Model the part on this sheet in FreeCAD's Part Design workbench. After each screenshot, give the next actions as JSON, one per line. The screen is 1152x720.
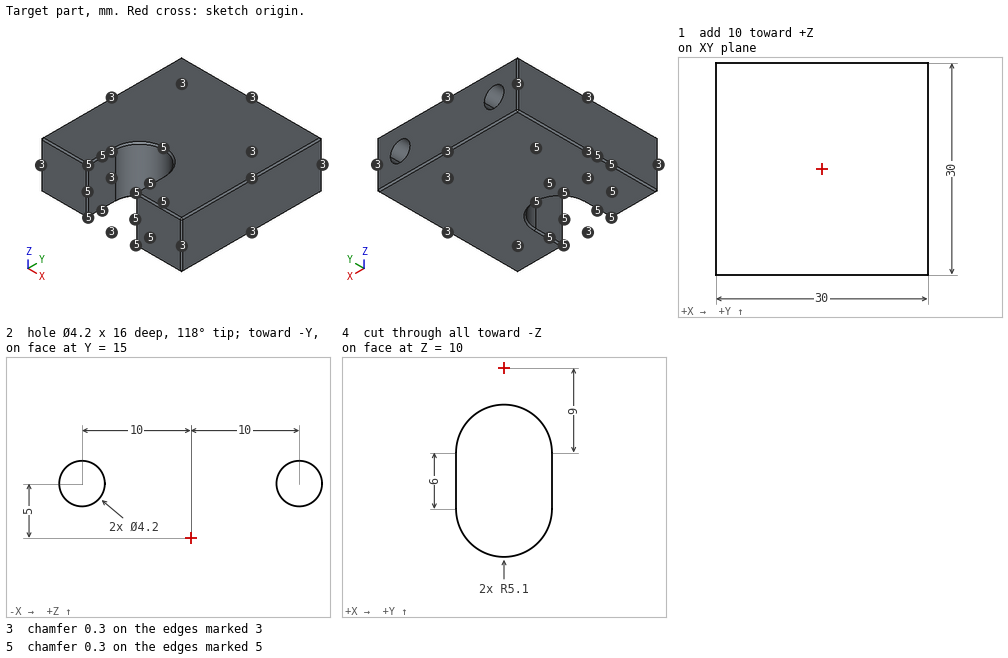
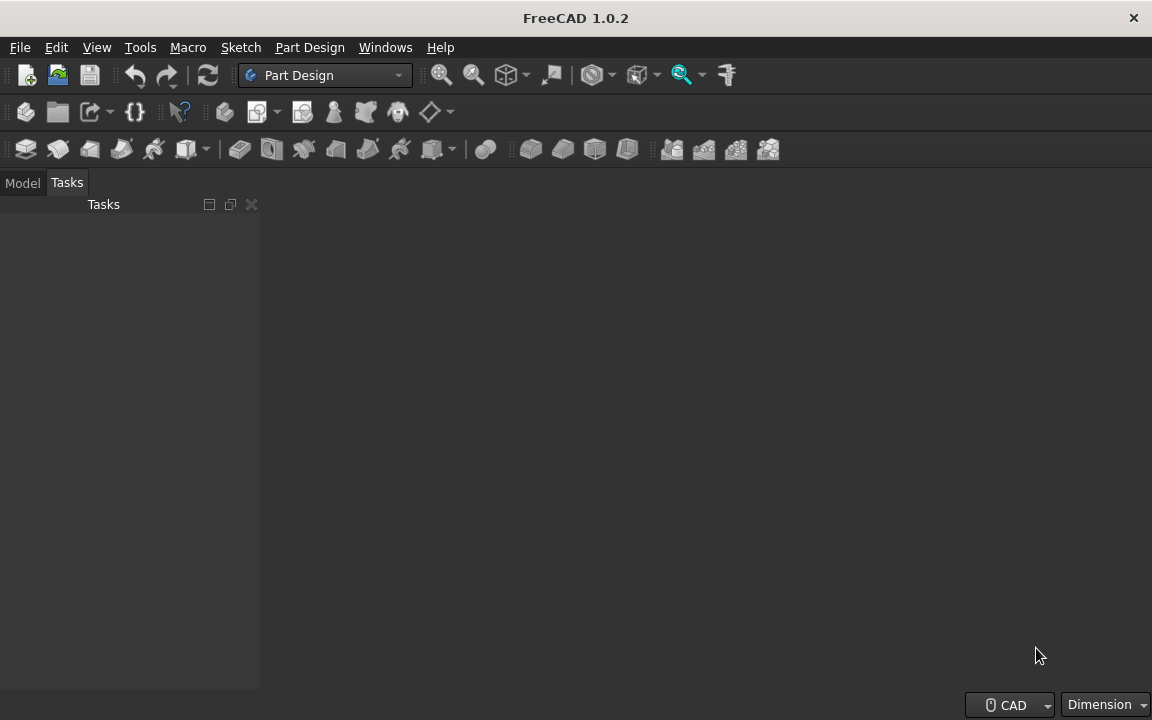
{"action": "left_click", "coordinate": [26, 76]}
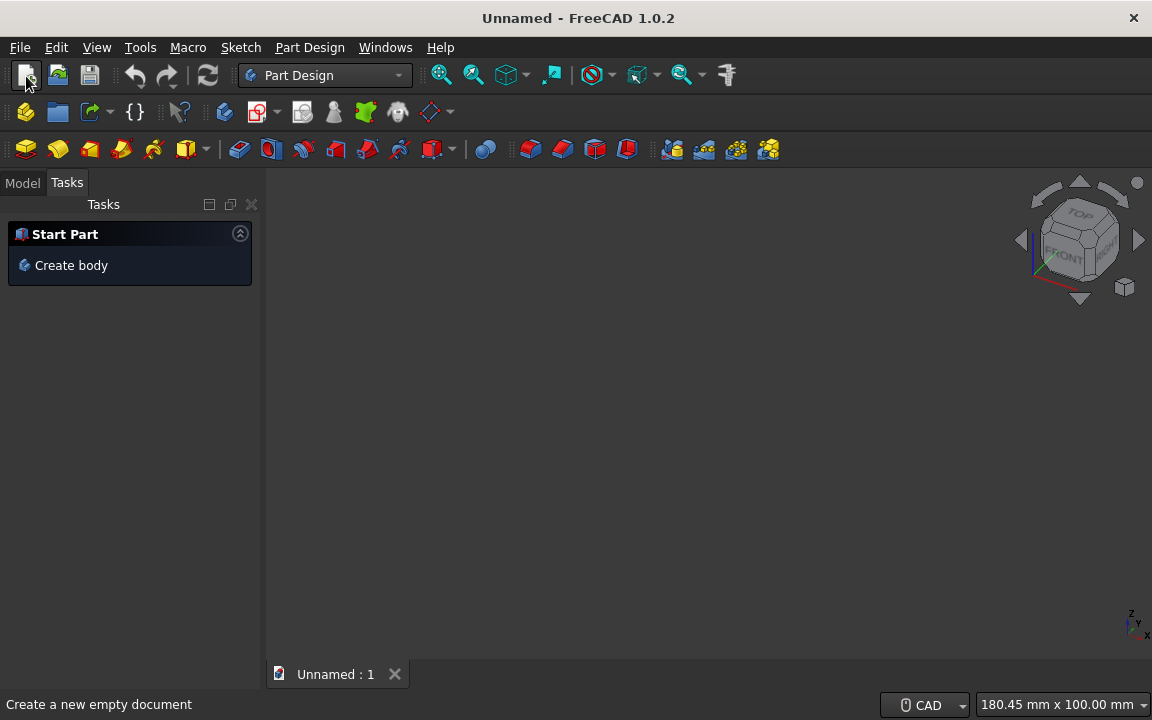
{"action": "left_click", "coordinate": [258, 112]}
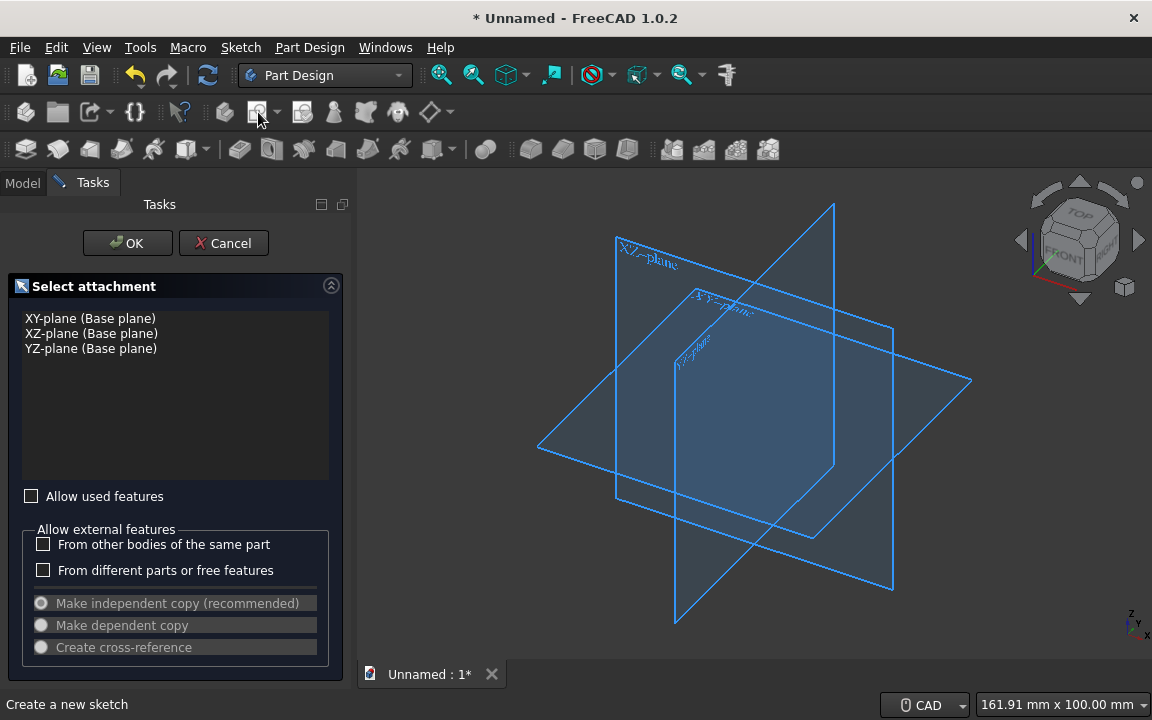
{"action": "left_click", "coordinate": [82, 318]}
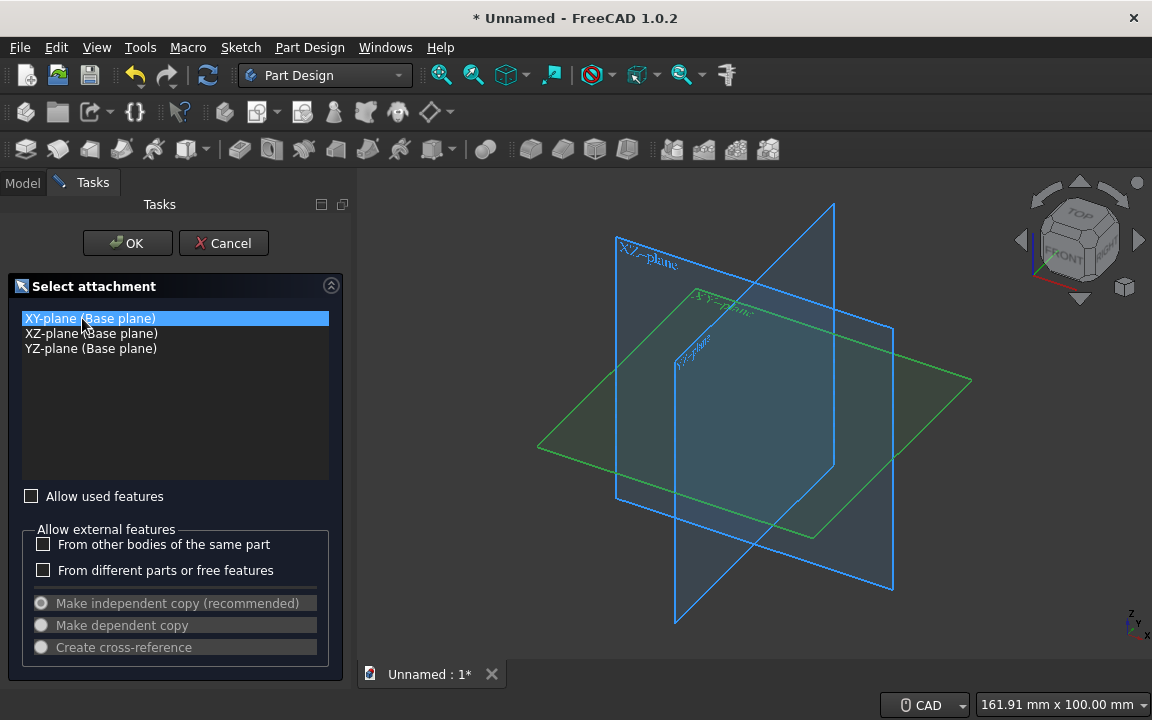
{"action": "left_click", "coordinate": [128, 243]}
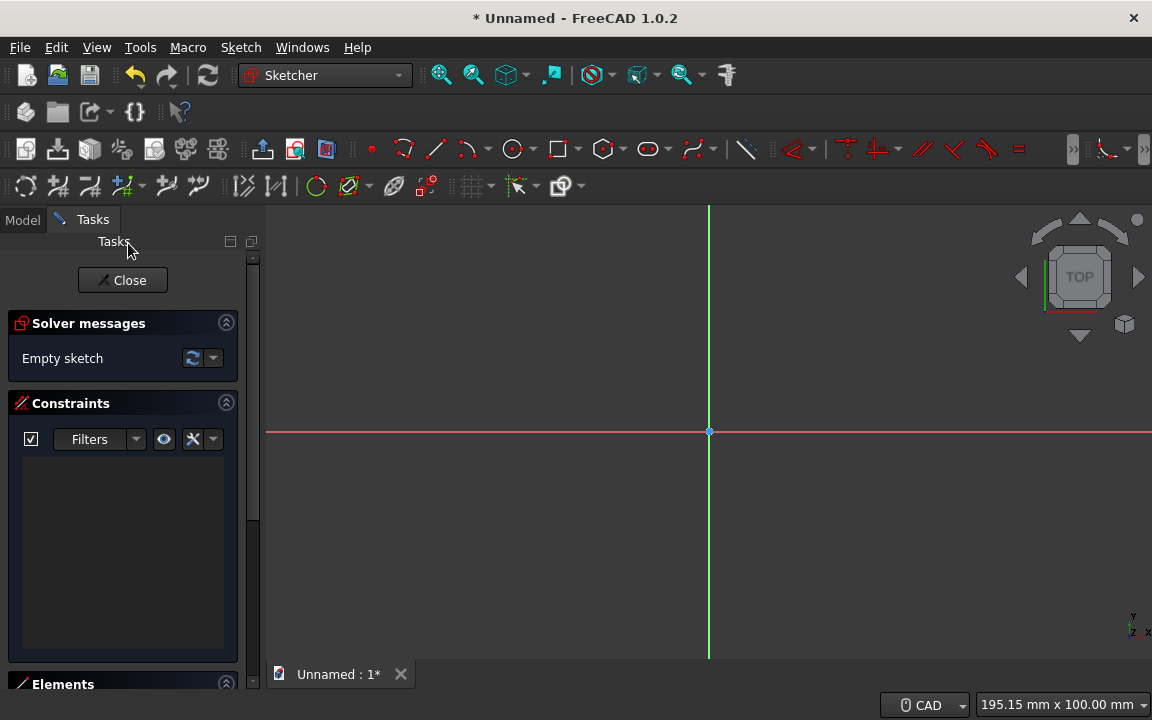
{"action": "scroll", "coordinate": [765, 432], "scroll_direction": "up", "scroll_amount": 4}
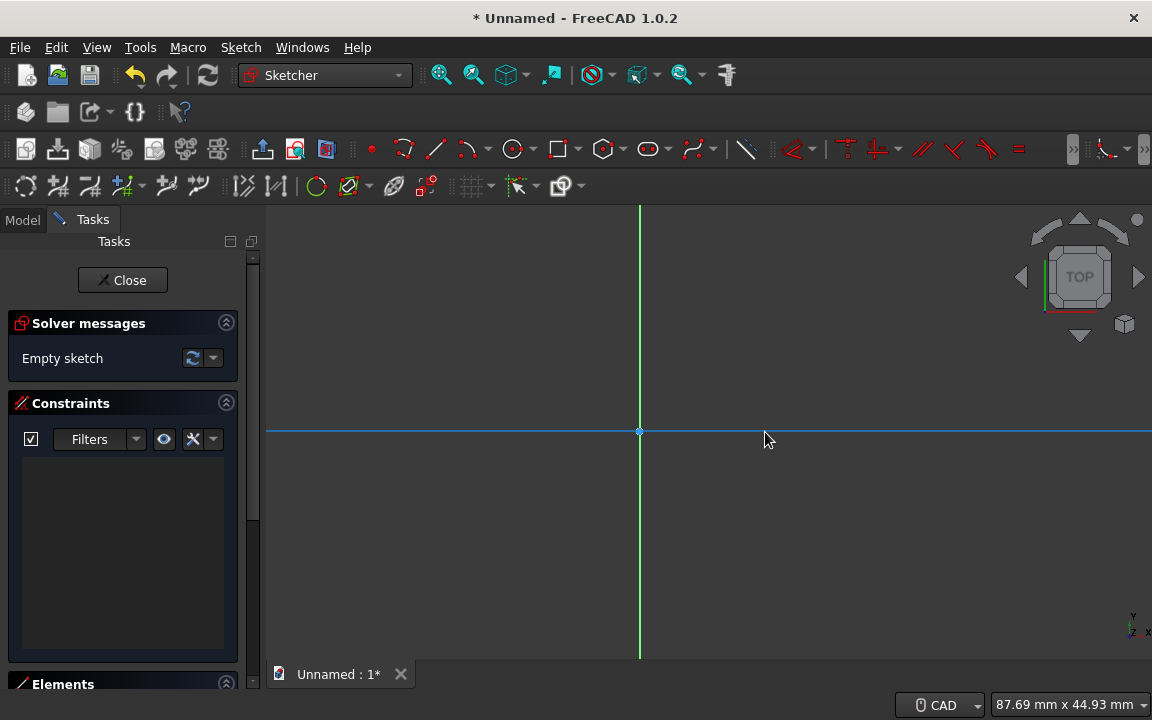
{"action": "left_click", "coordinate": [580, 150]}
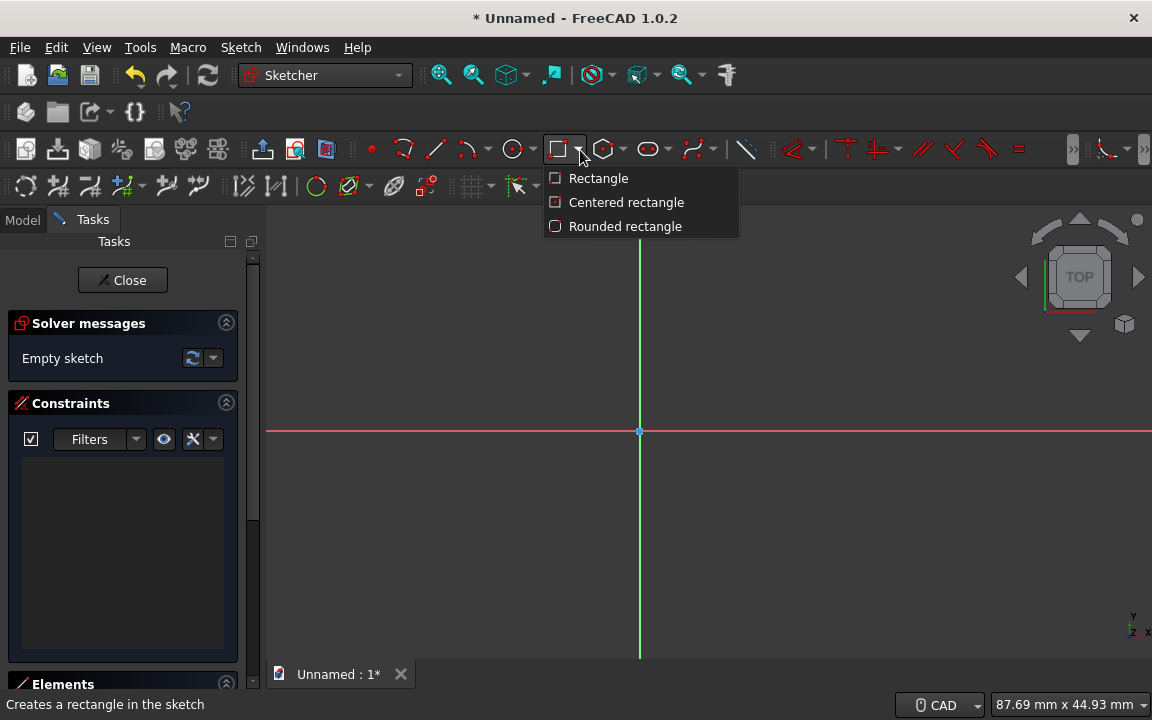
{"action": "left_click", "coordinate": [642, 202]}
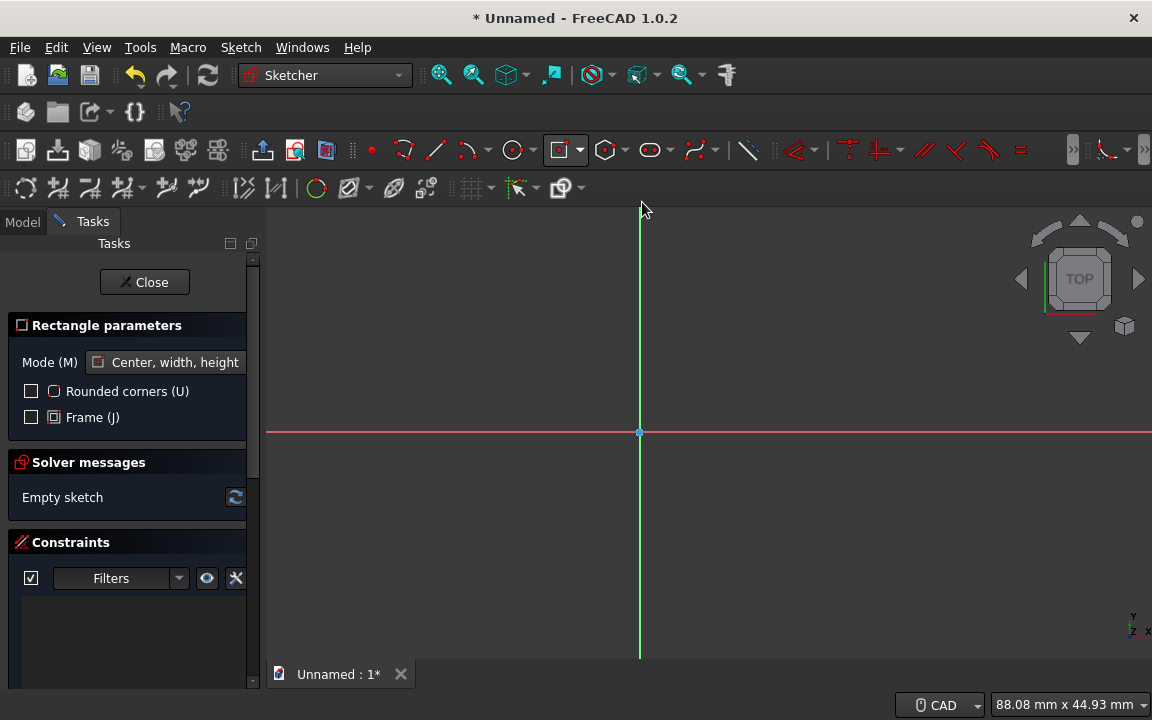
{"action": "left_click", "coordinate": [640, 432]}
{"action": "left_click", "coordinate": [791, 281]}
{"action": "key", "text": "Escape"}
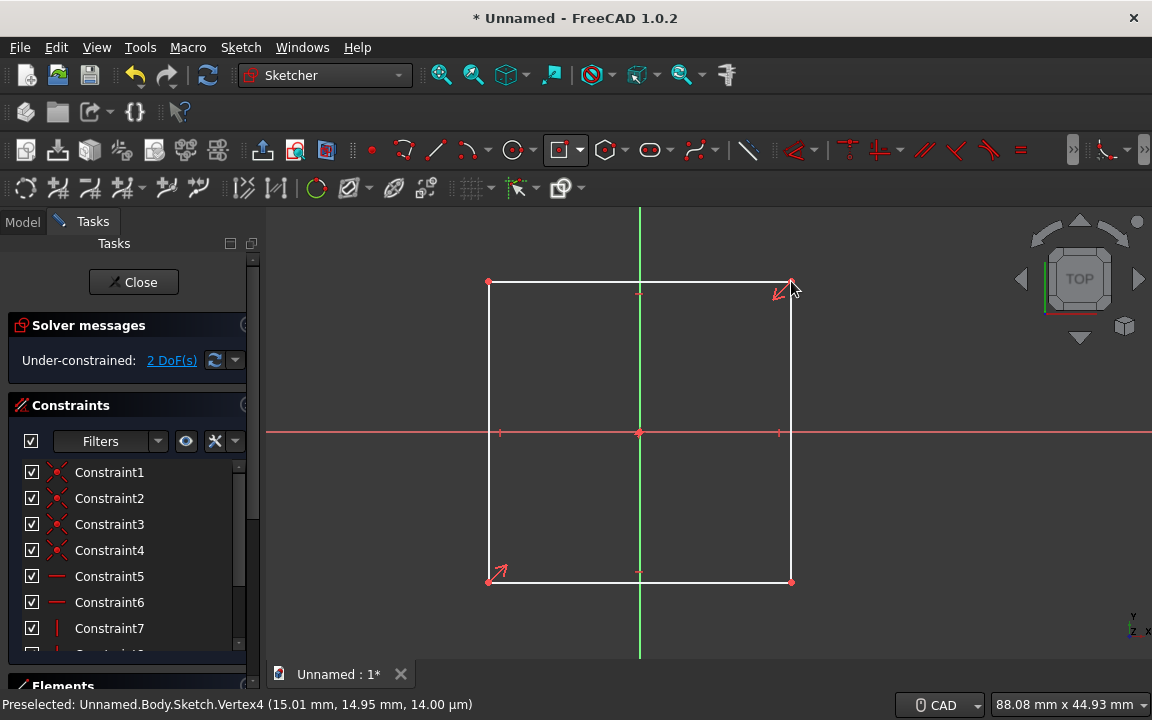
{"action": "left_click", "coordinate": [794, 150]}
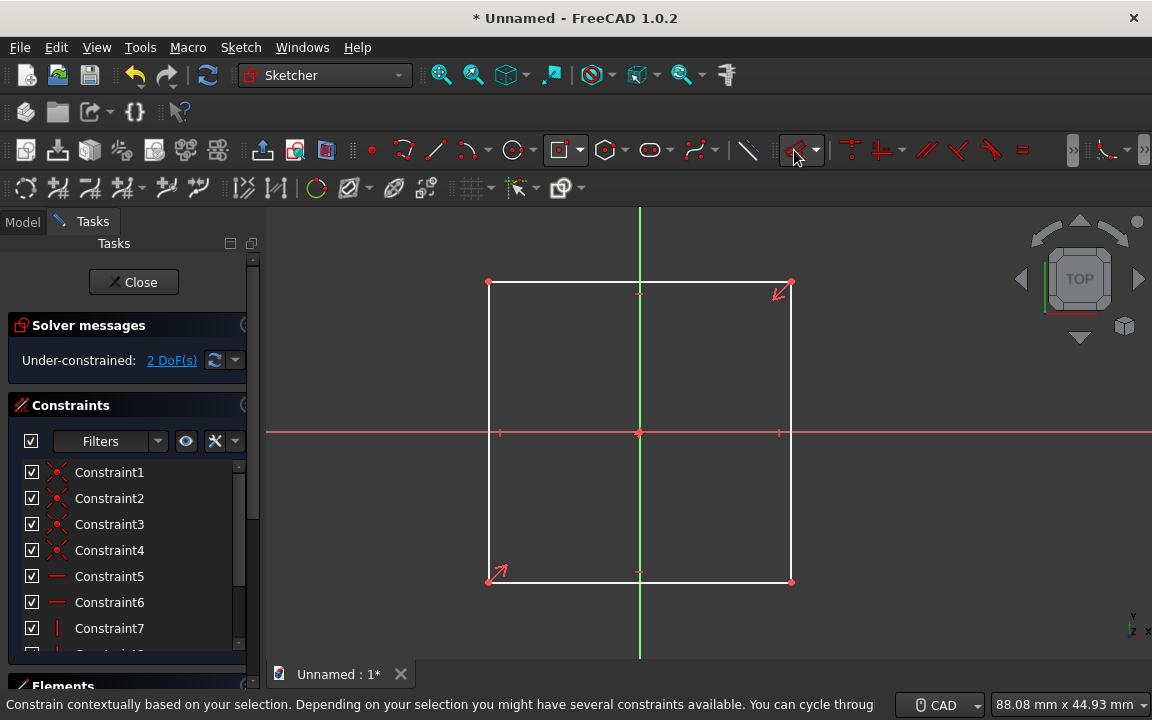
{"action": "left_click", "coordinate": [580, 583]}
{"action": "left_click", "coordinate": [571, 617]}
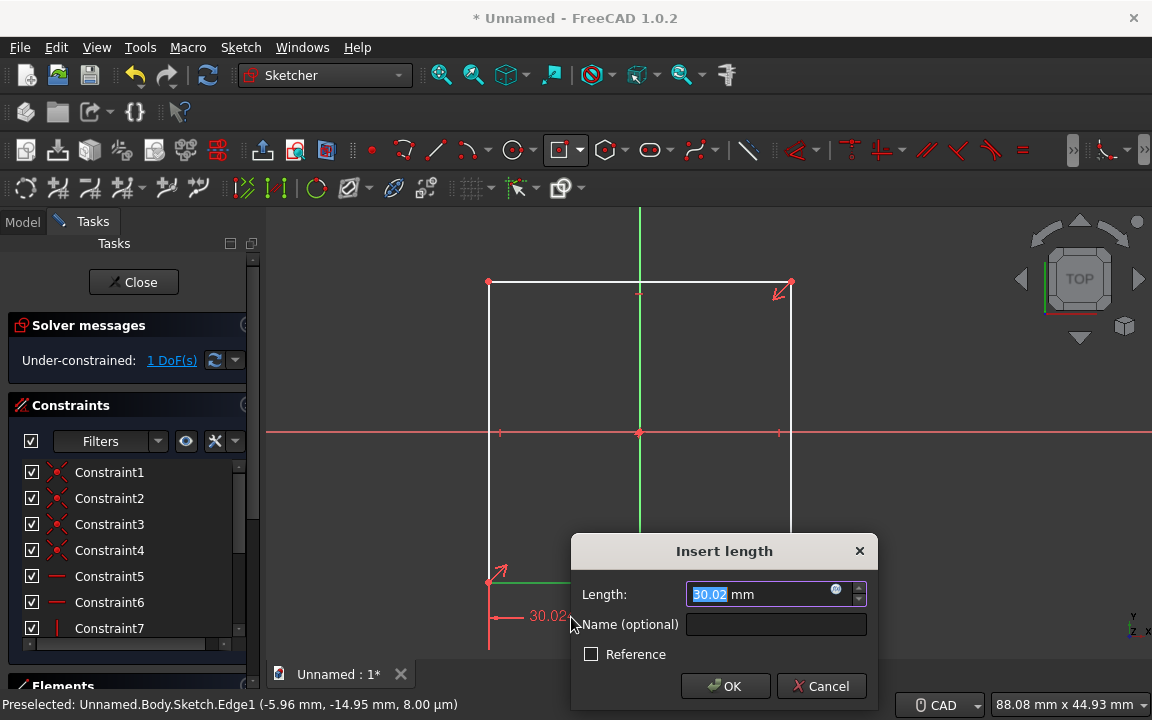
{"action": "type", "text": "30"}
{"action": "key", "text": "Return"}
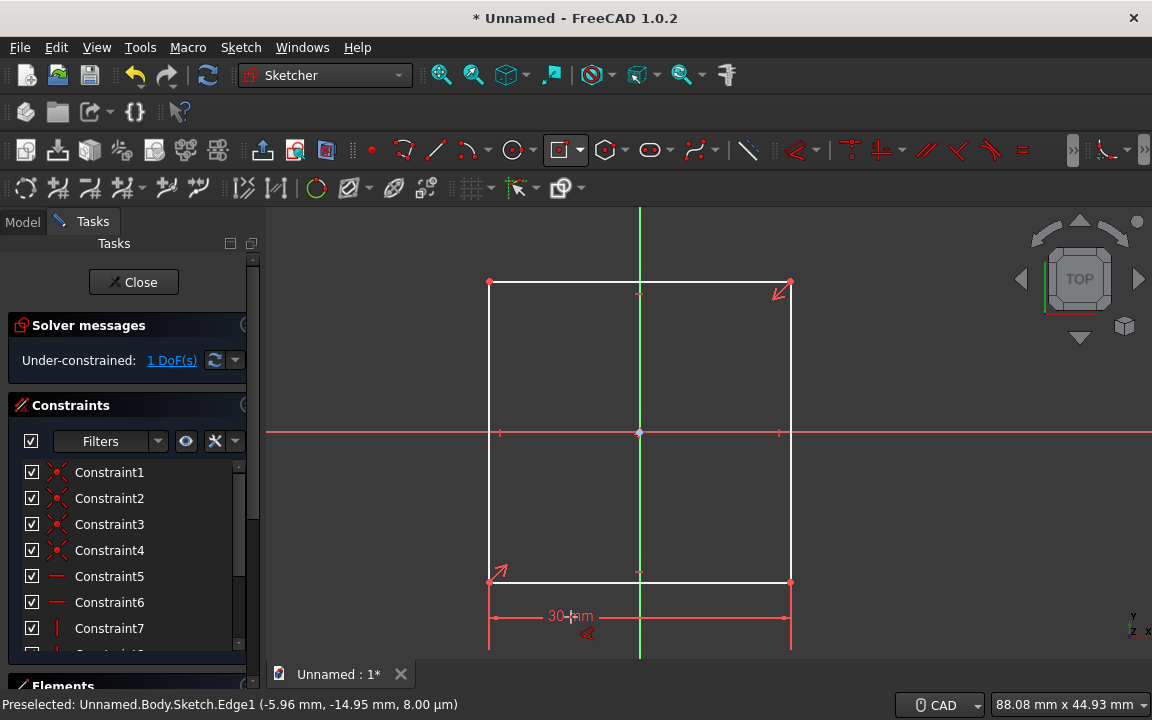
{"action": "left_click", "coordinate": [791, 493]}
{"action": "left_click", "coordinate": [825, 363]}